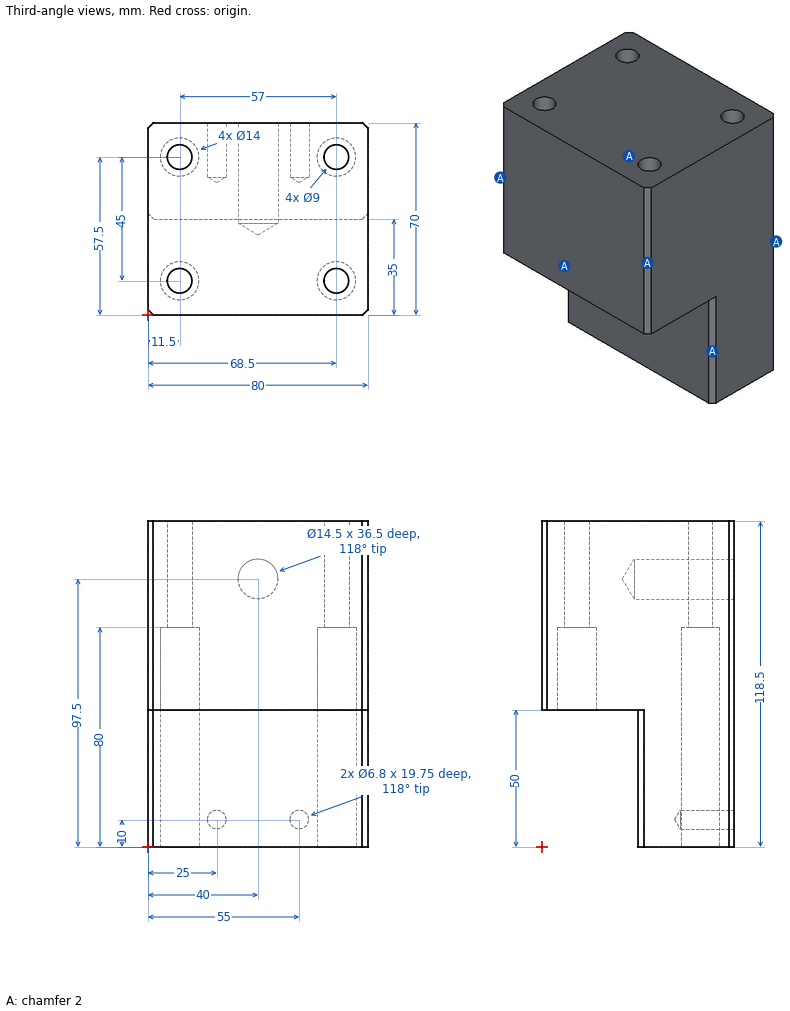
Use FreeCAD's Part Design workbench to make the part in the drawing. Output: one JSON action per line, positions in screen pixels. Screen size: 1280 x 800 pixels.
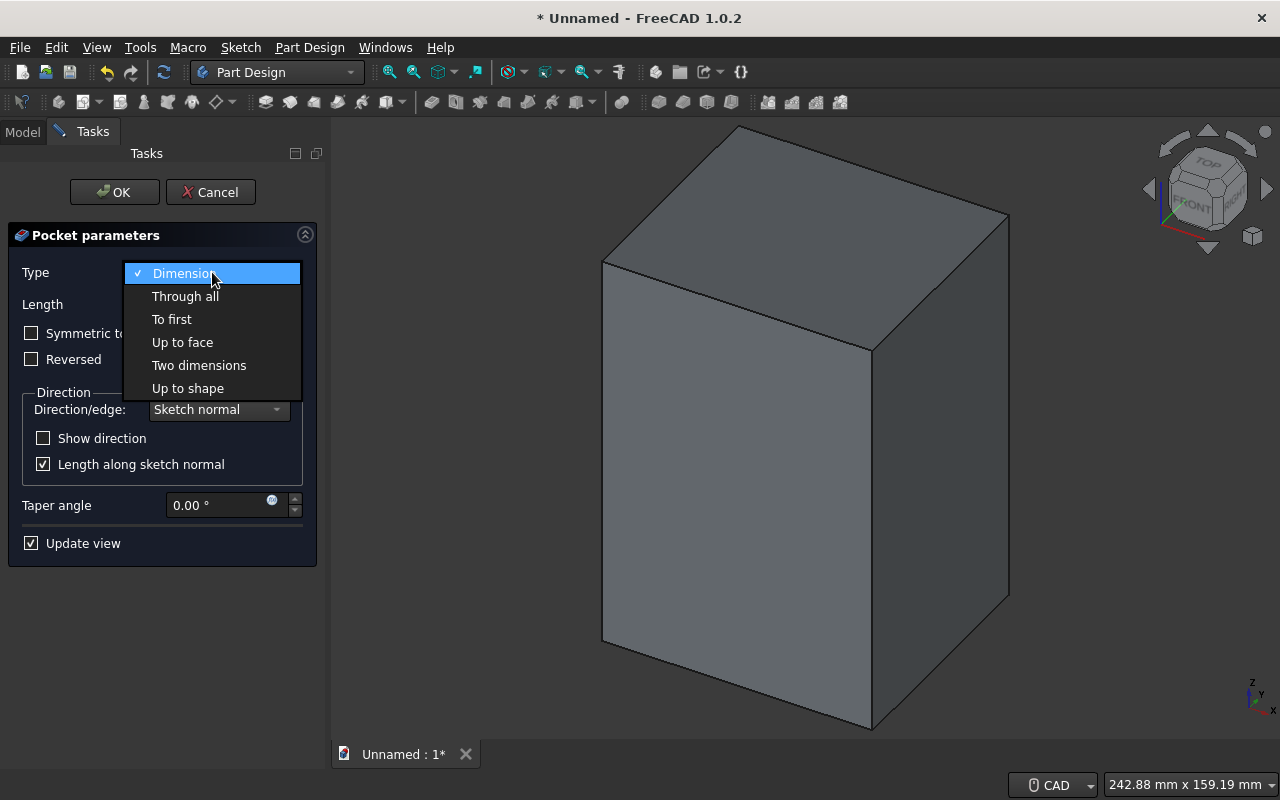
{"action": "left_click", "coordinate": [212, 296]}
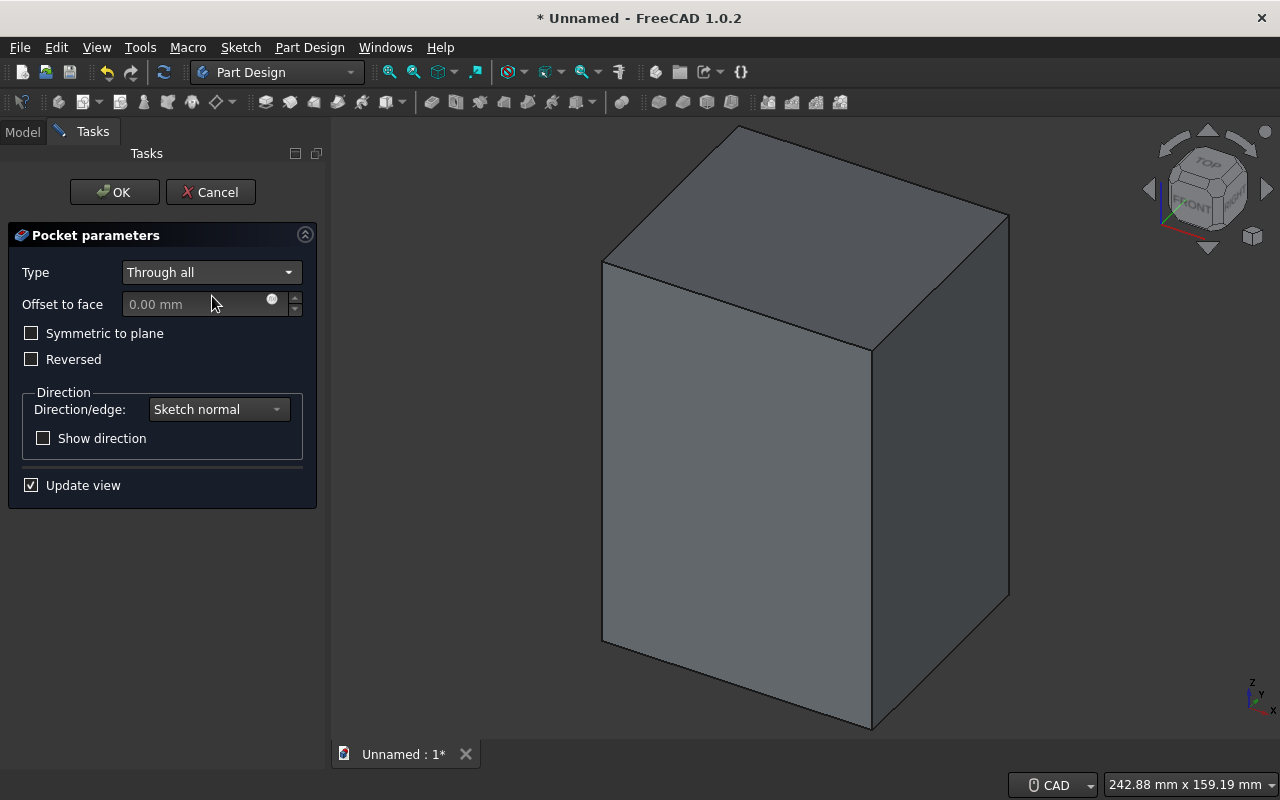
{"action": "left_click", "coordinate": [30, 359]}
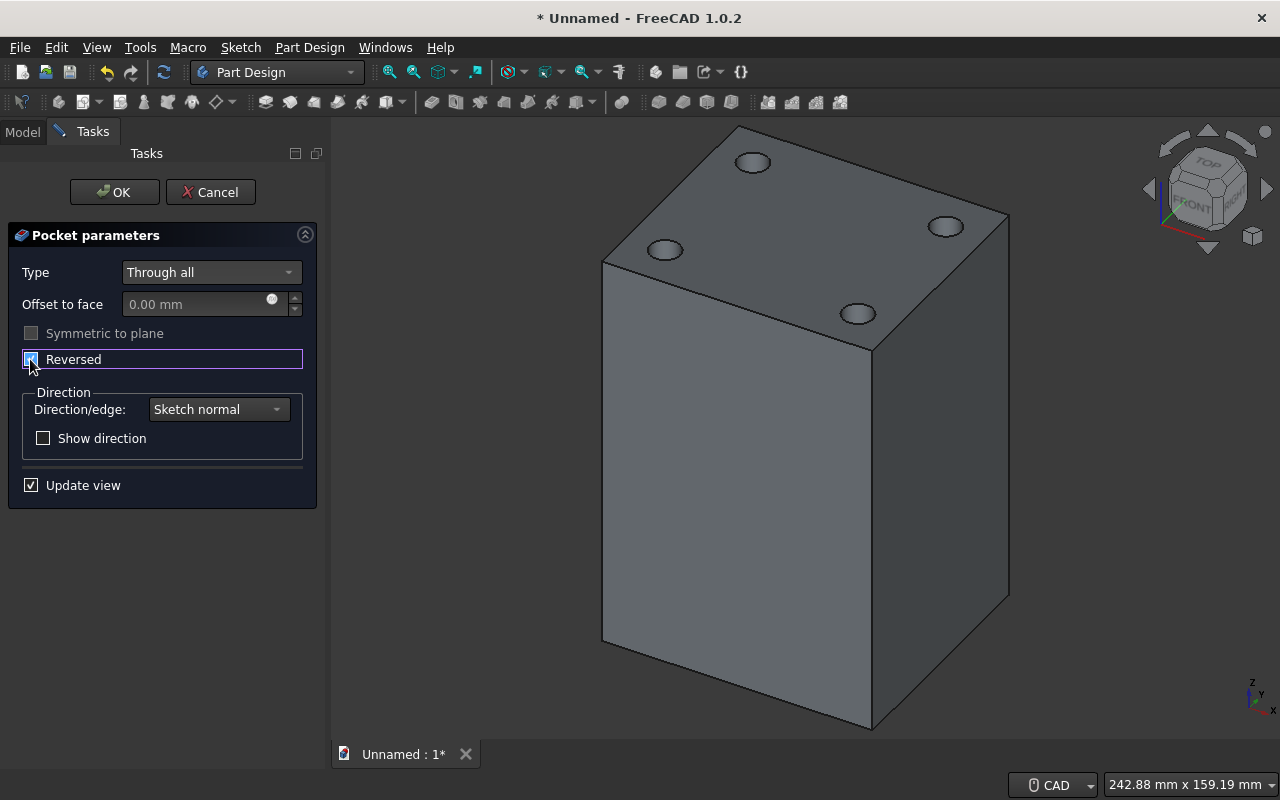
{"action": "left_click", "coordinate": [115, 192]}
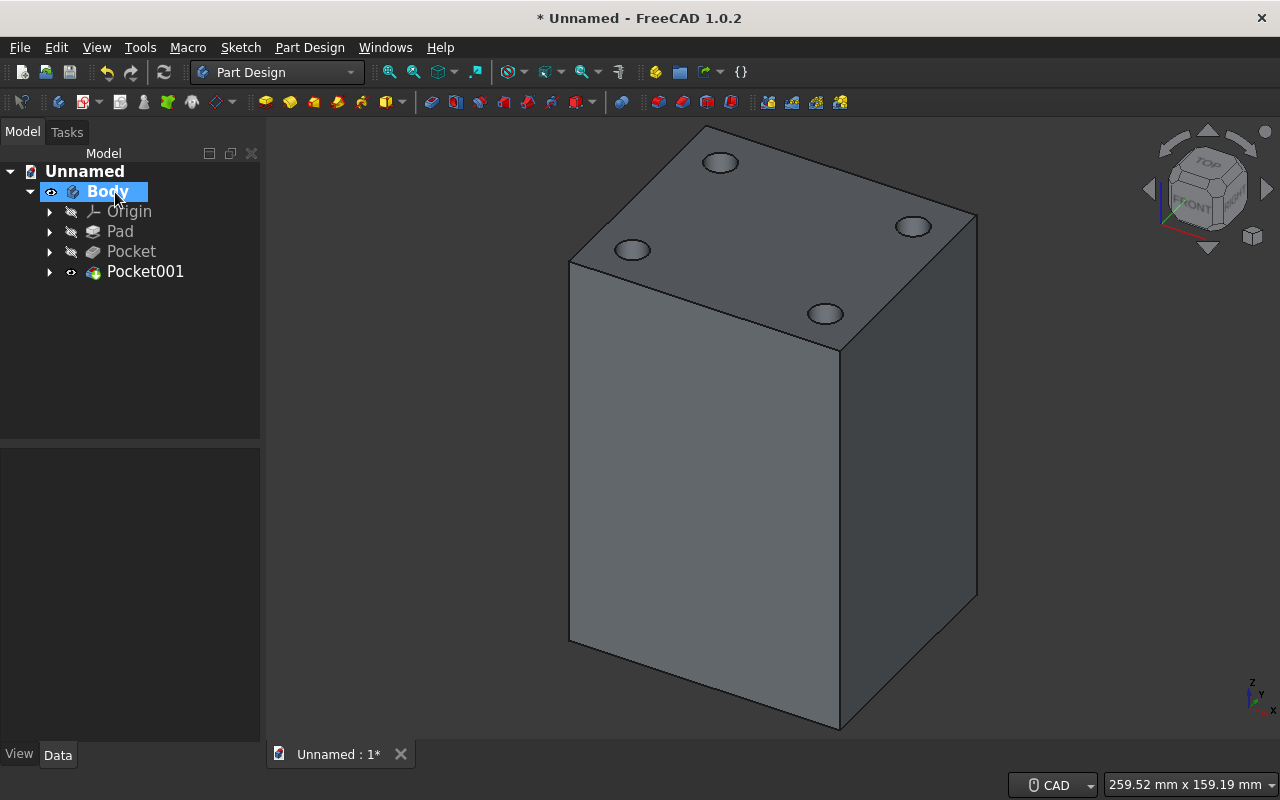
{"action": "left_click", "coordinate": [84, 102]}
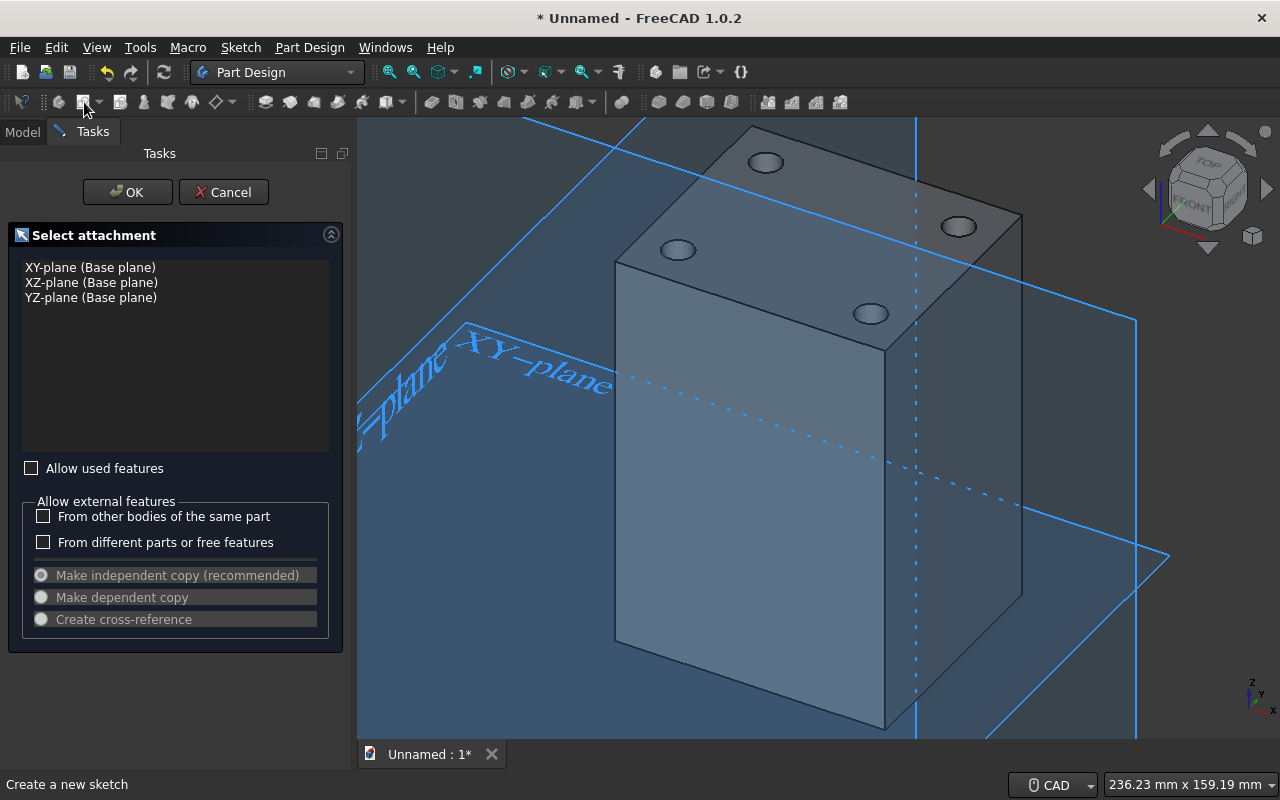
{"action": "left_click", "coordinate": [82, 268]}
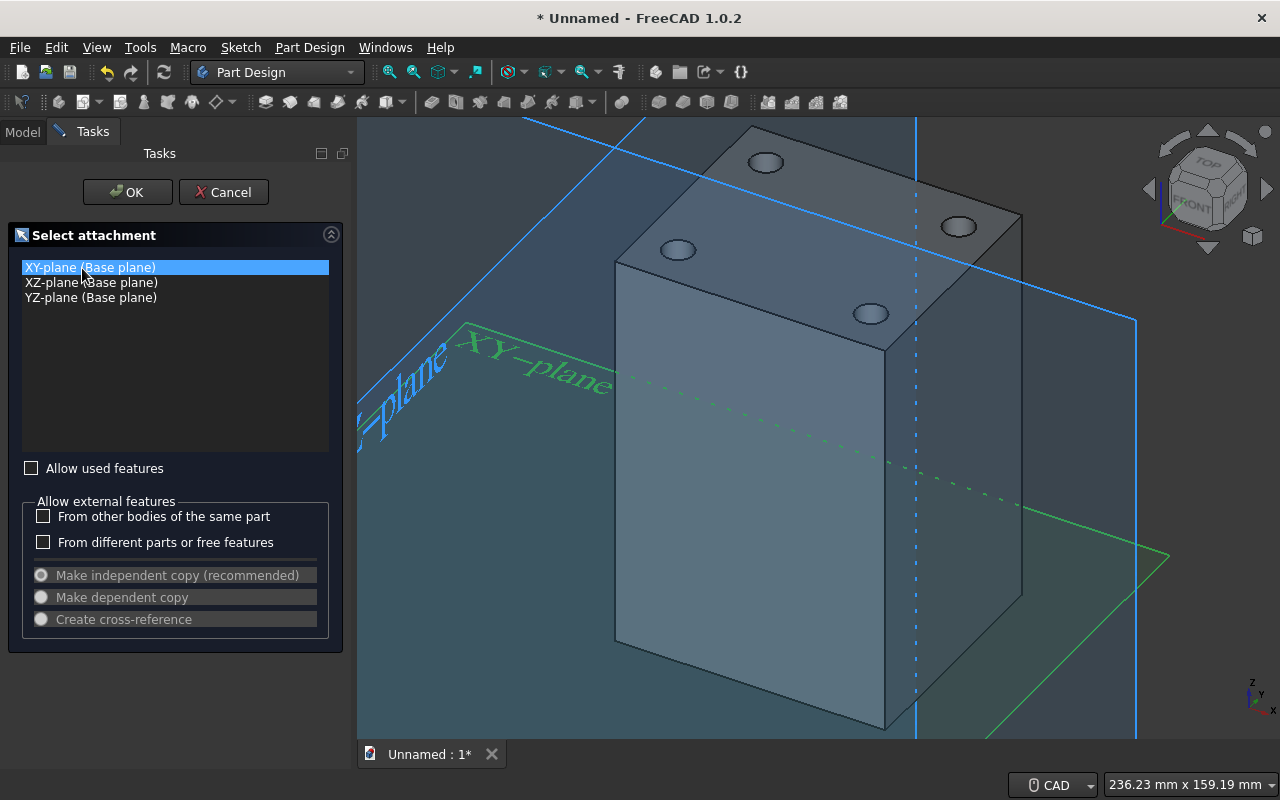
{"action": "left_click", "coordinate": [128, 192]}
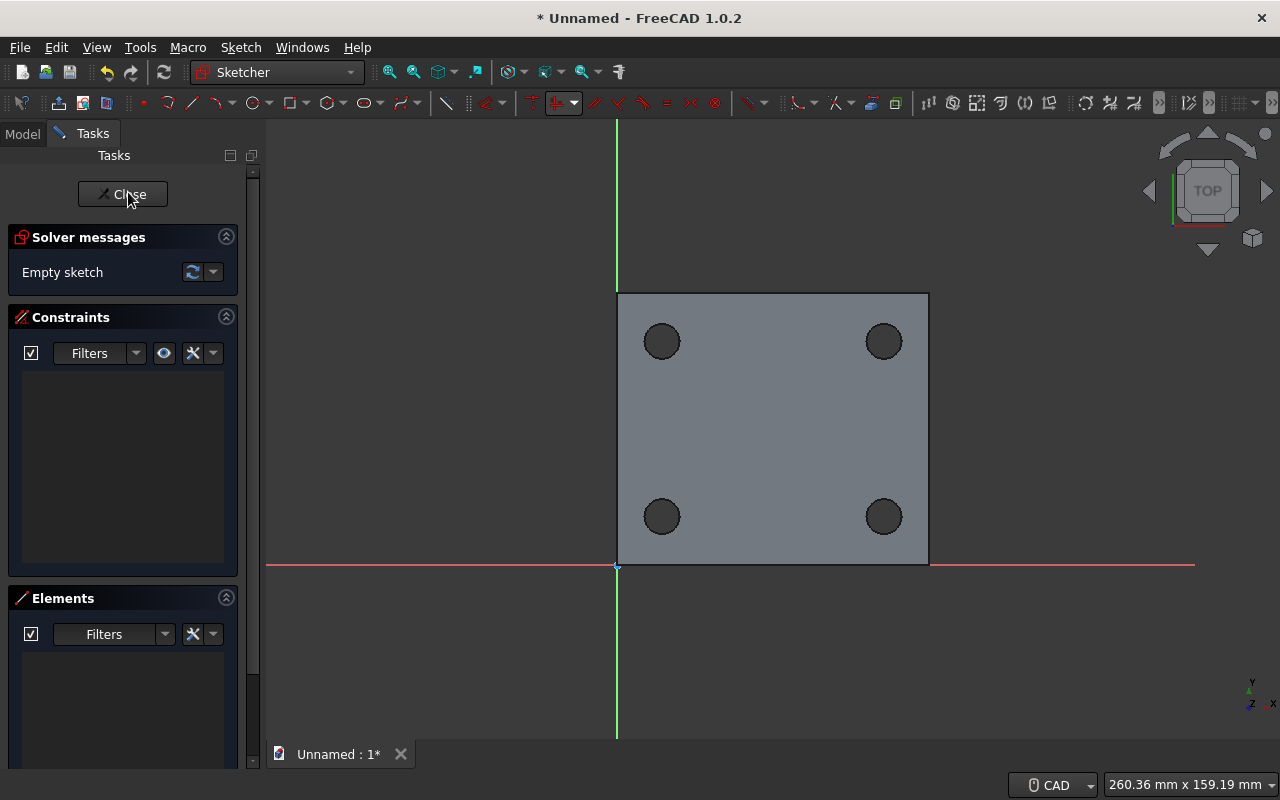
{"action": "key", "text": "q s"}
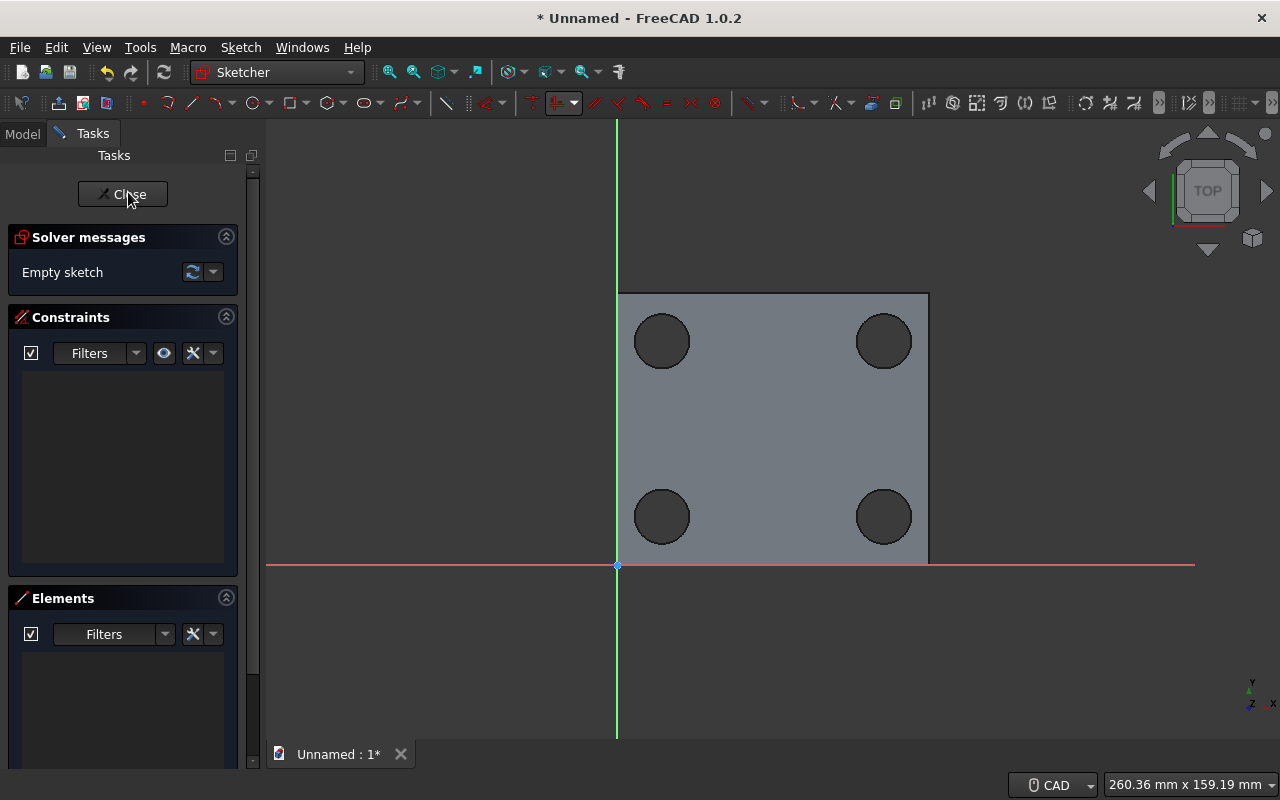
{"action": "scroll", "coordinate": [856, 580], "scroll_direction": "up", "scroll_amount": 3}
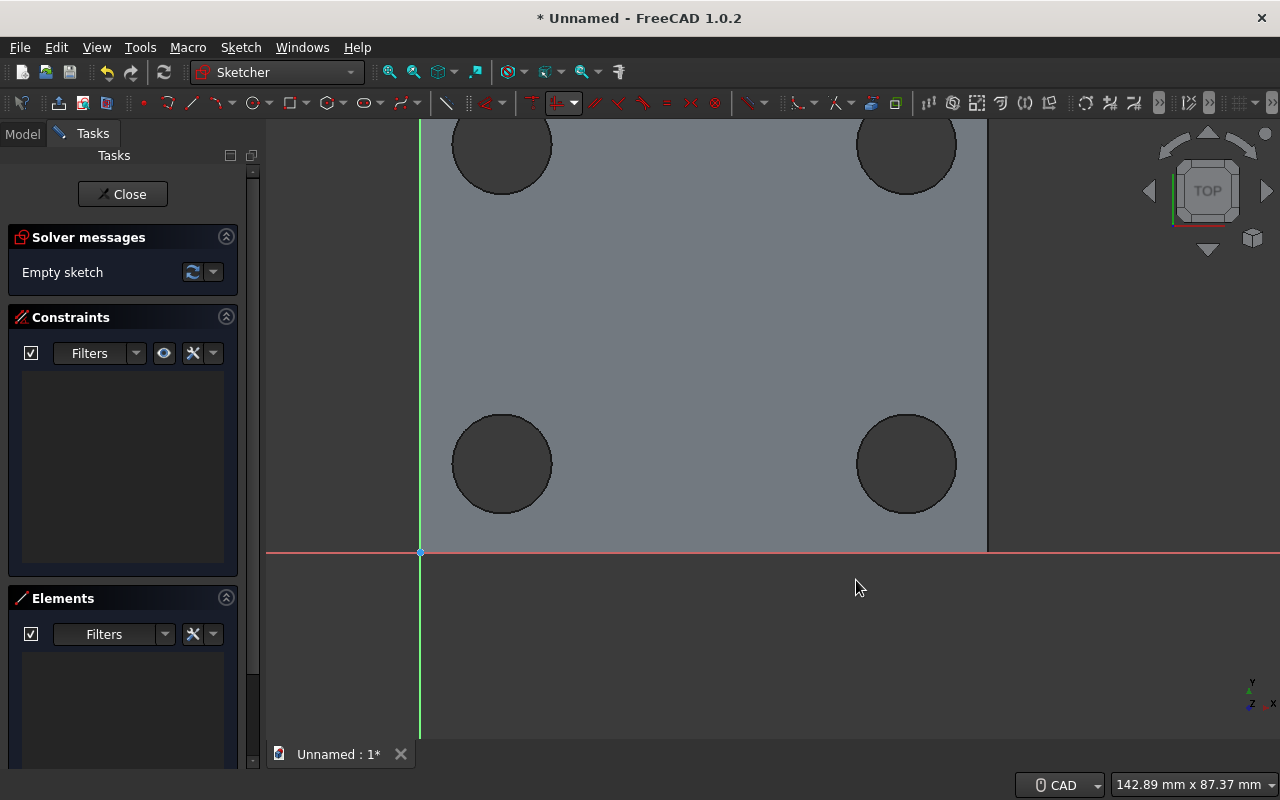
{"action": "key", "text": "g r"}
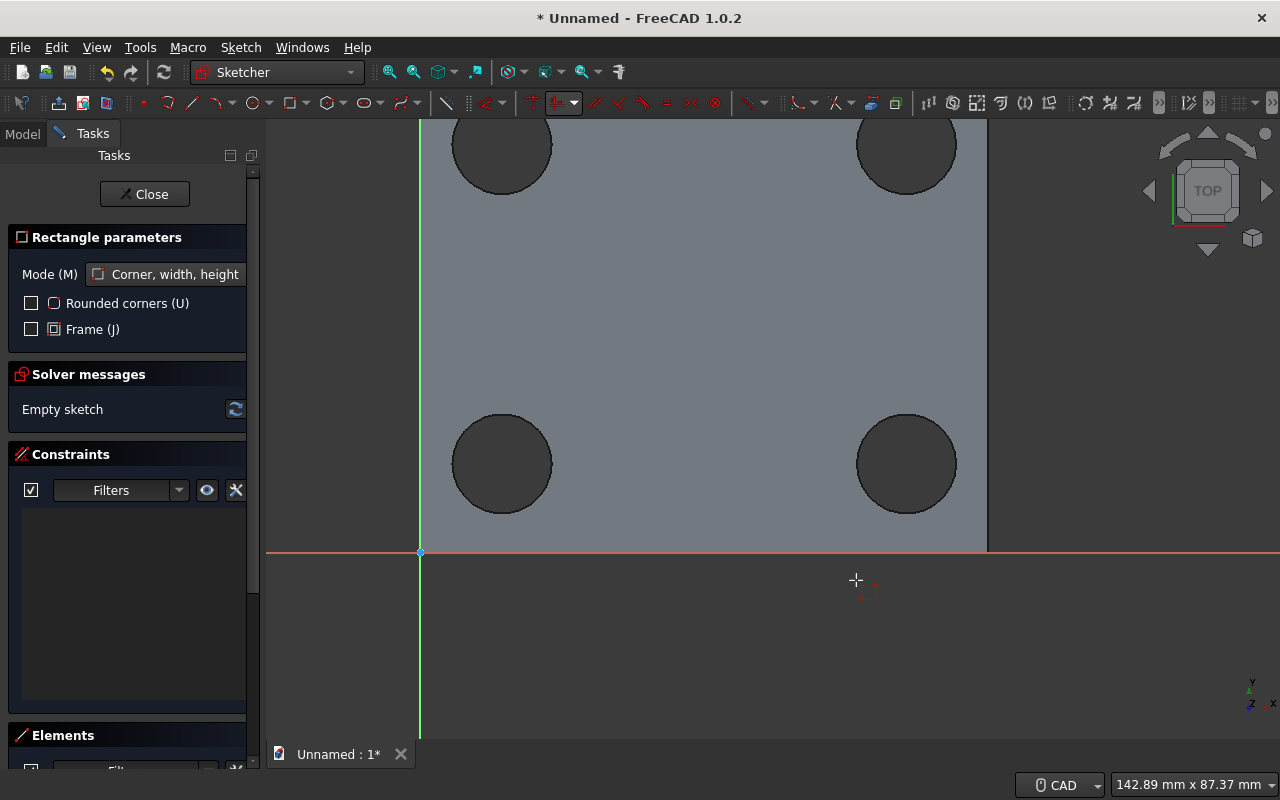
{"action": "left_click", "coordinate": [420, 553]}
{"action": "left_click", "coordinate": [988, 304]}
{"action": "key", "text": "Escape"}